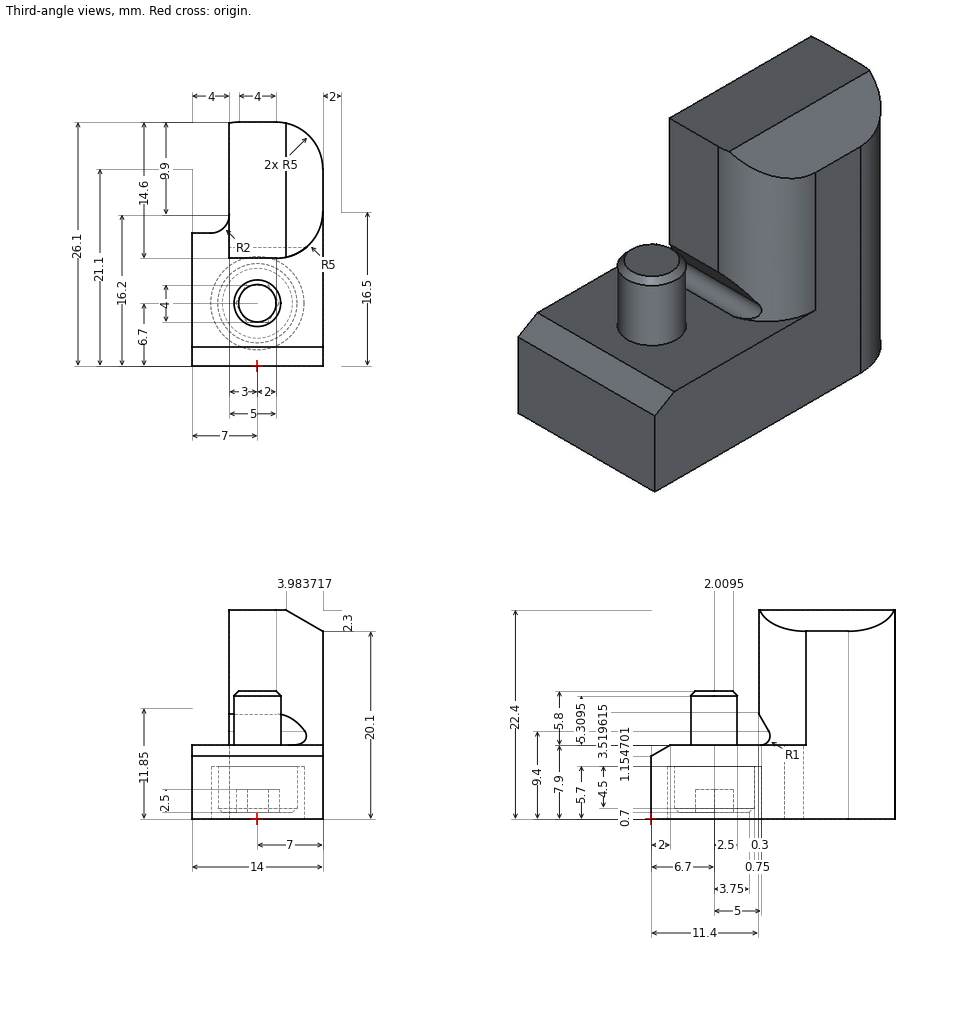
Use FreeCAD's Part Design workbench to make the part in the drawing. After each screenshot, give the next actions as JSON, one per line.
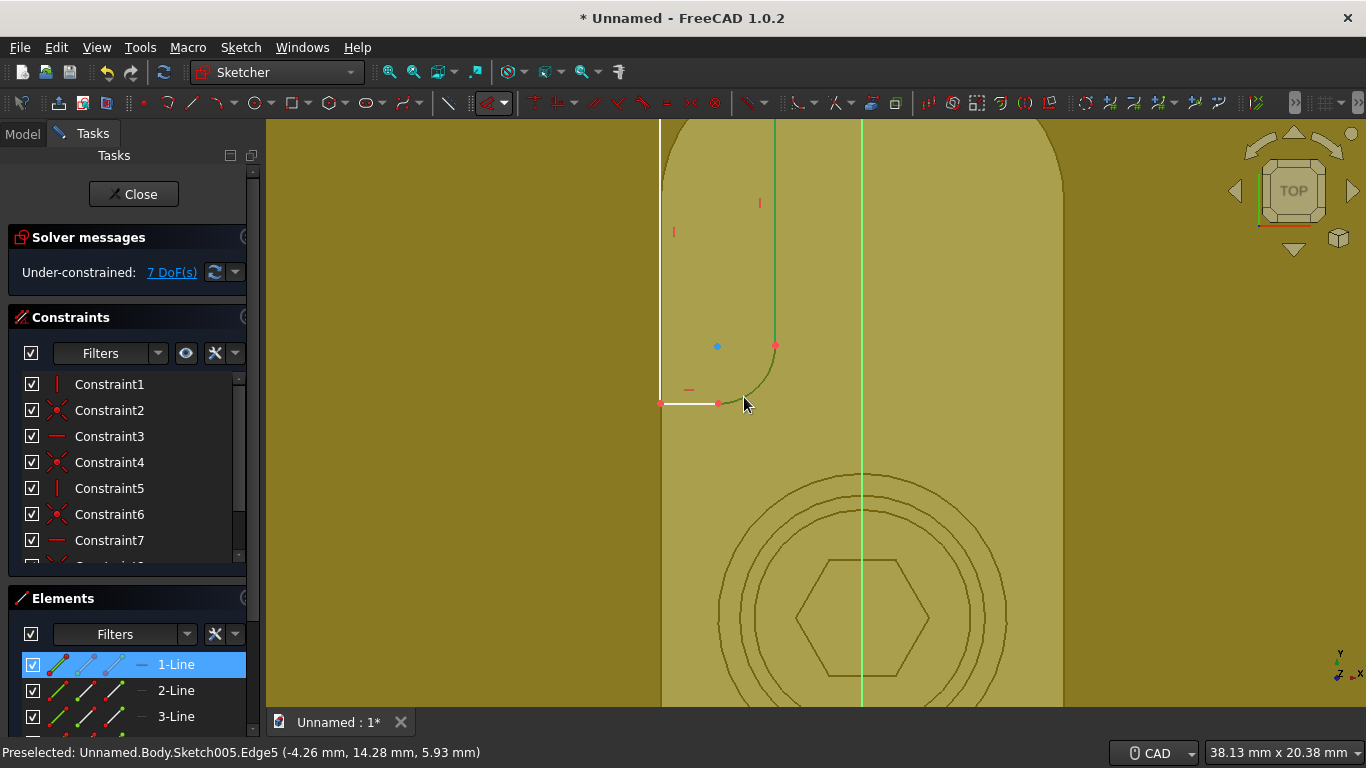
{"action": "left_click", "coordinate": [644, 104]}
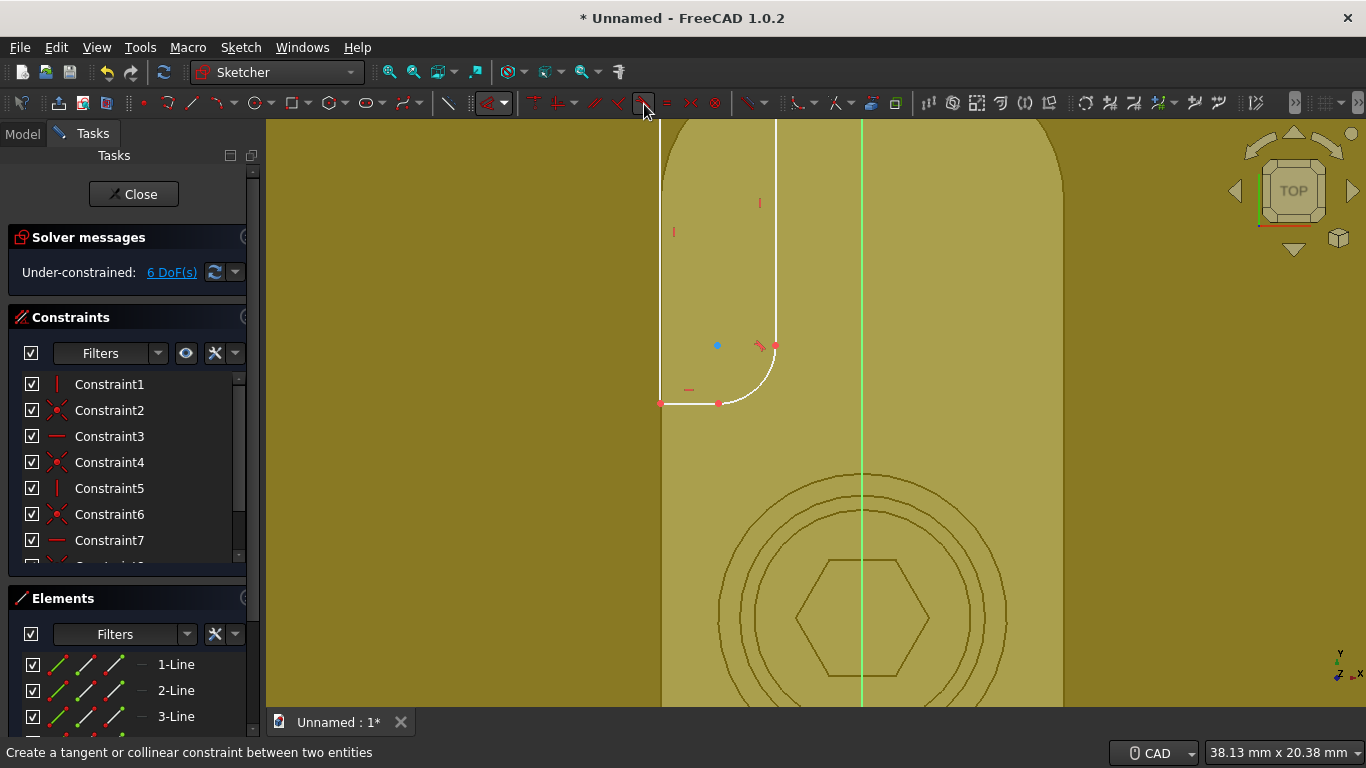
{"action": "left_click", "coordinate": [678, 404]}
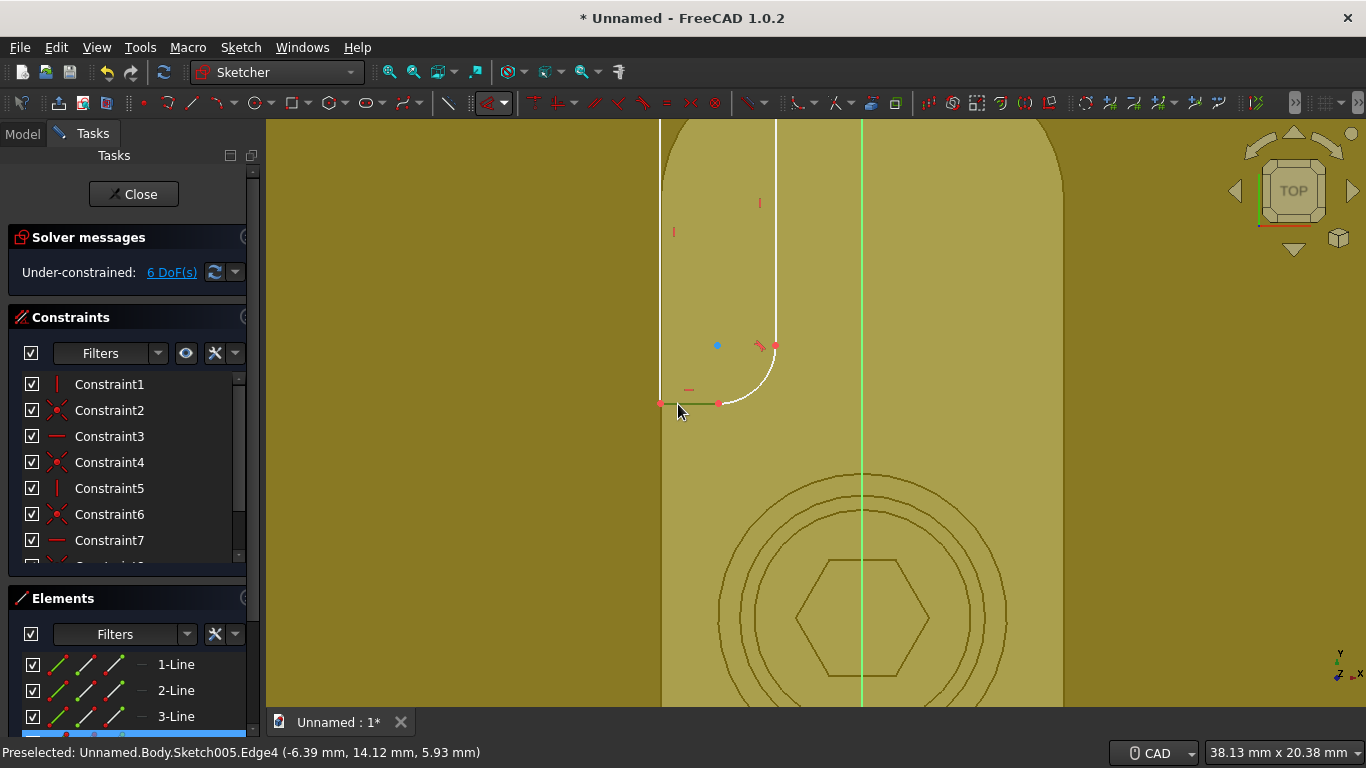
{"action": "left_click", "coordinate": [745, 397]}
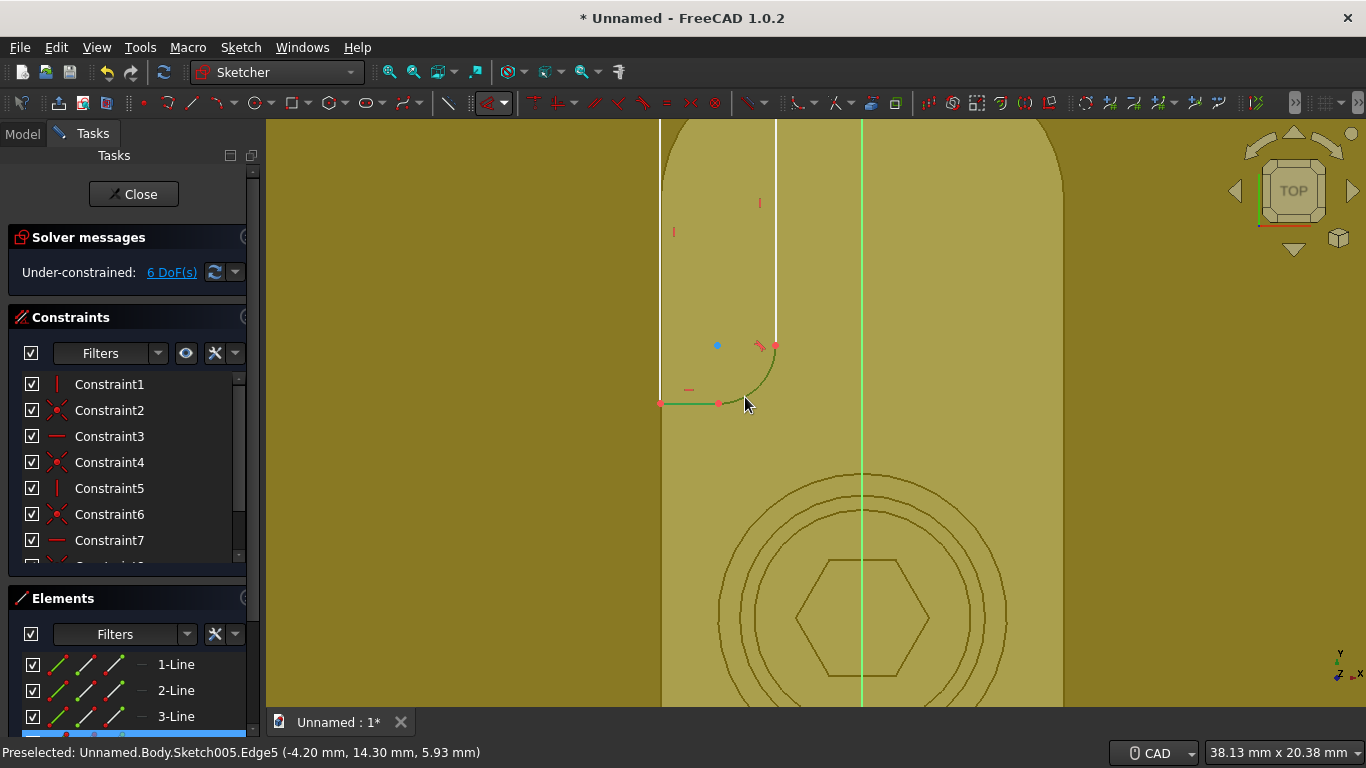
{"action": "left_click", "coordinate": [644, 104]}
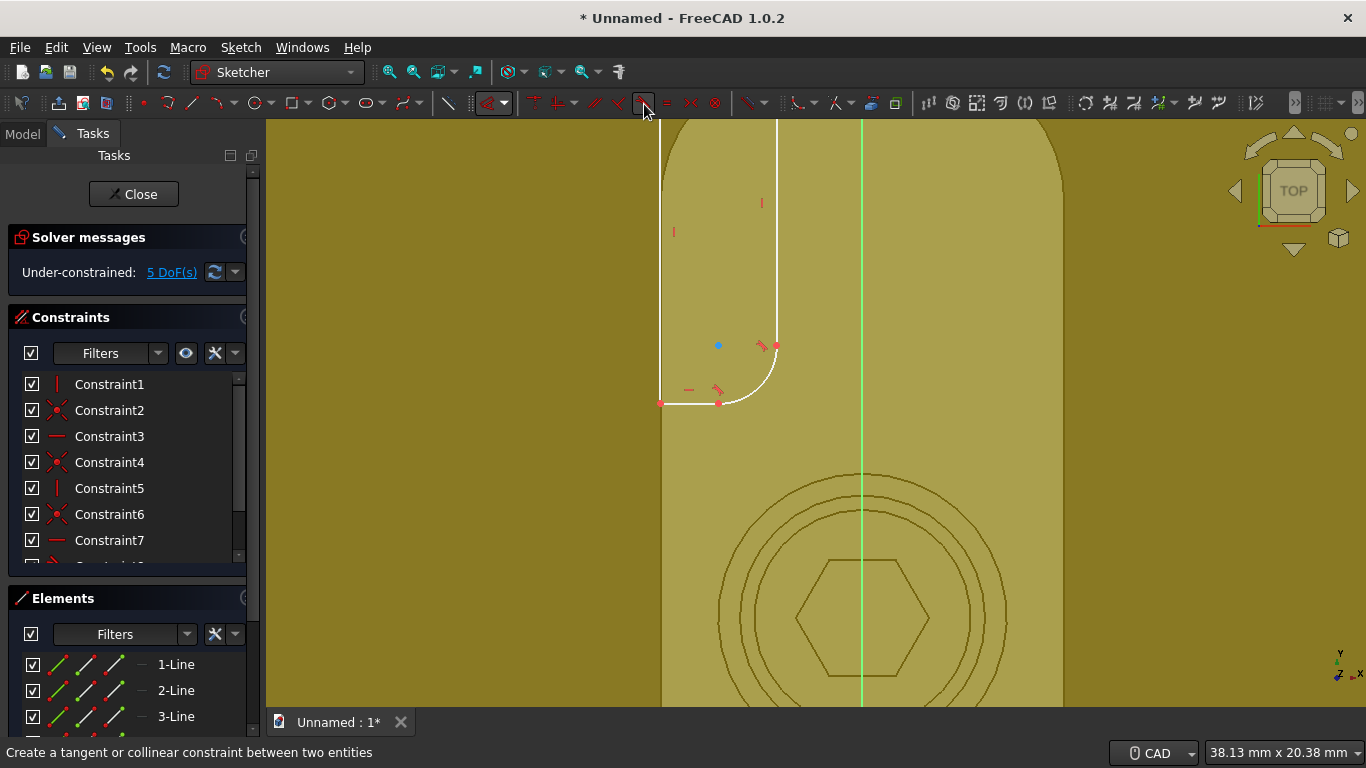
{"action": "left_click", "coordinate": [745, 397]}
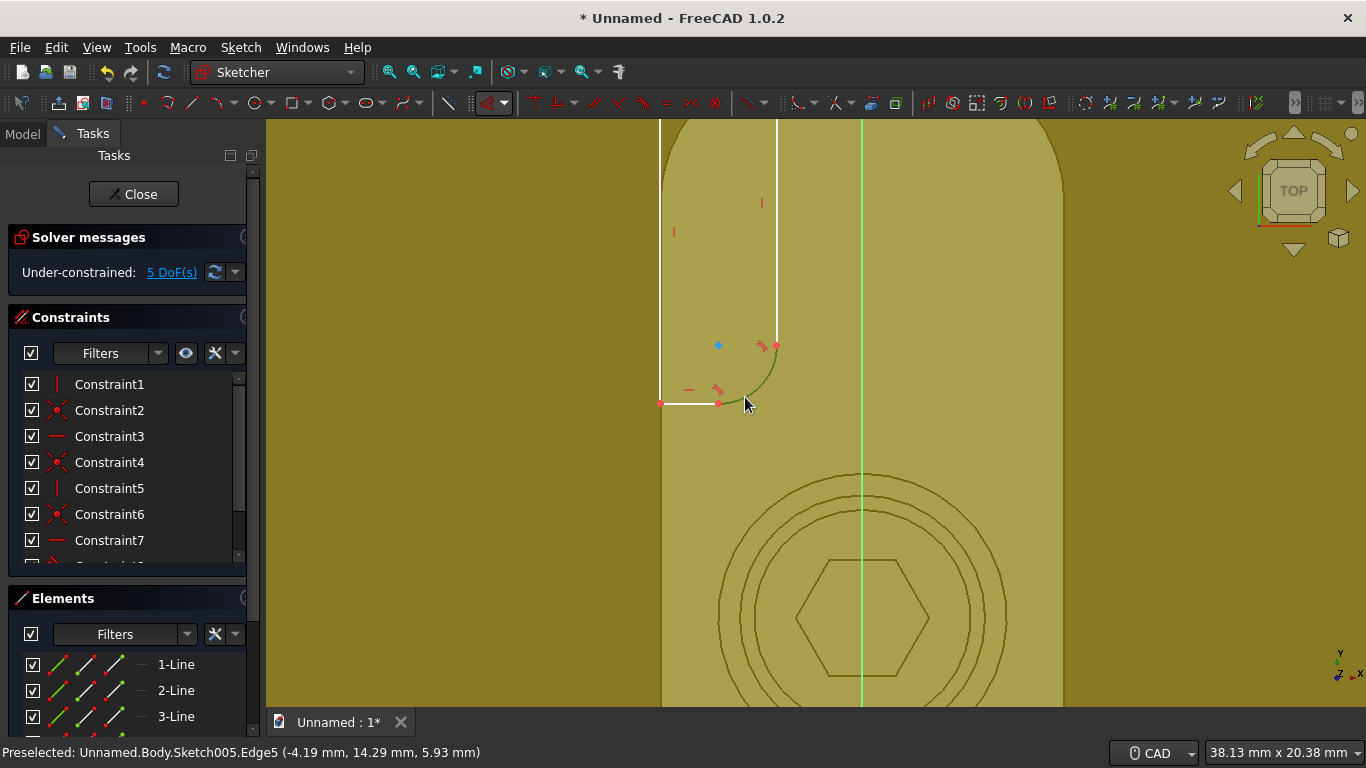
{"action": "left_click", "coordinate": [506, 104]}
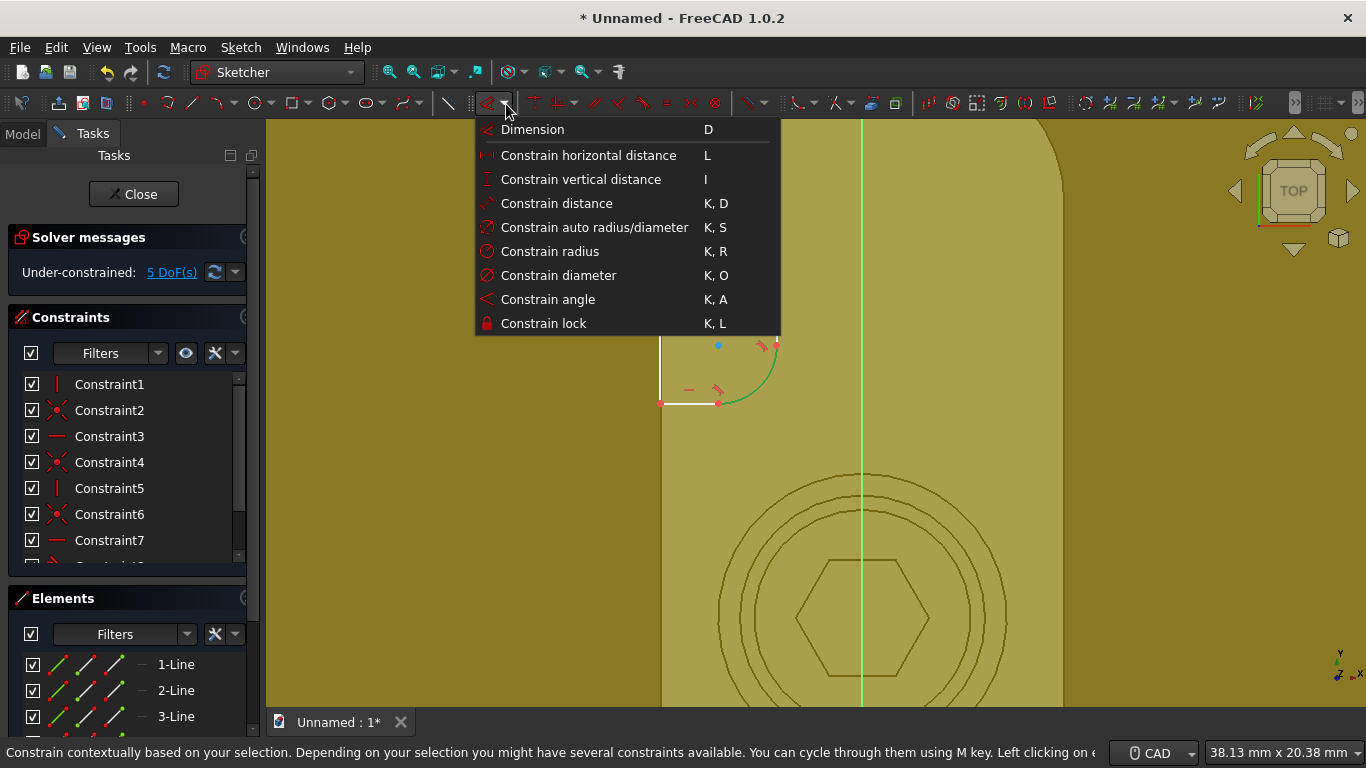
{"action": "left_click", "coordinate": [628, 251]}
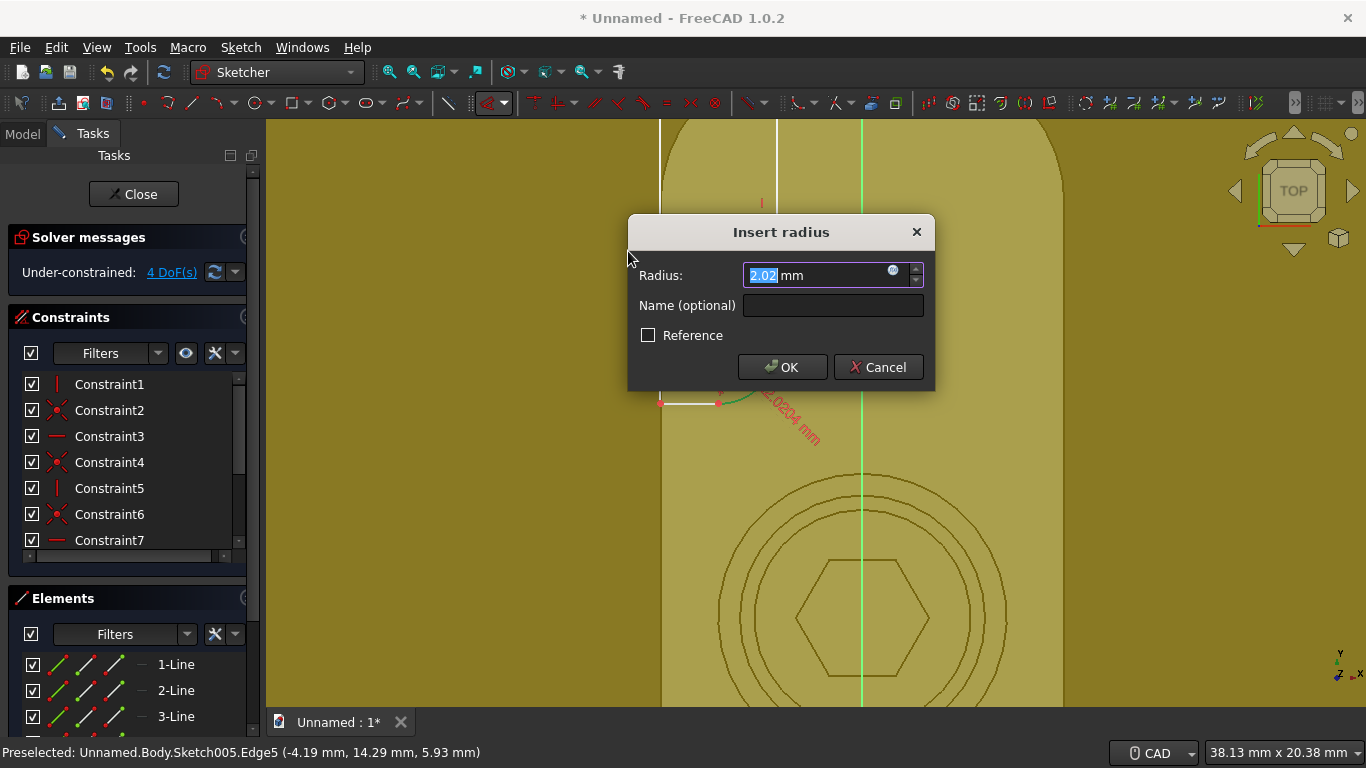
{"action": "type", "text": "2"}
{"action": "key", "text": "Return"}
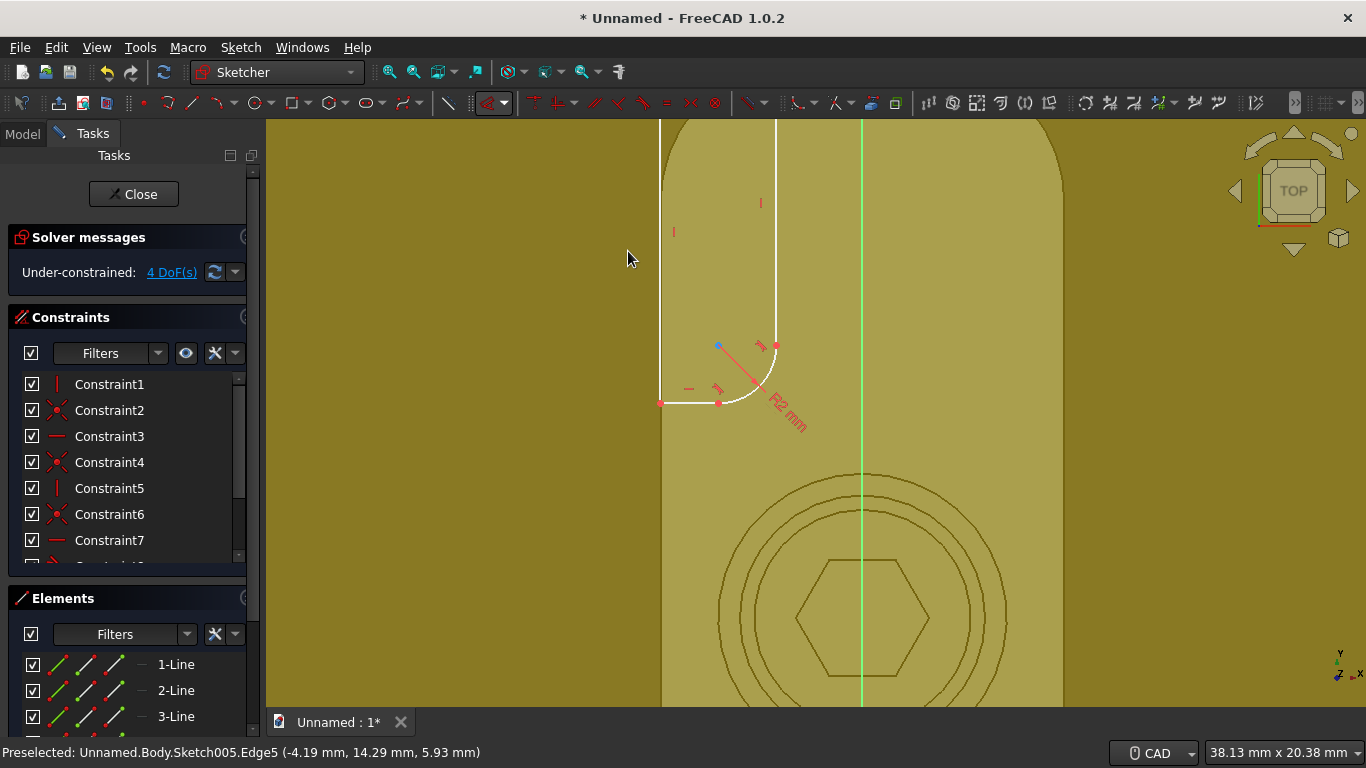
{"action": "scroll", "coordinate": [730, 386], "scroll_direction": "down", "scroll_amount": 3}